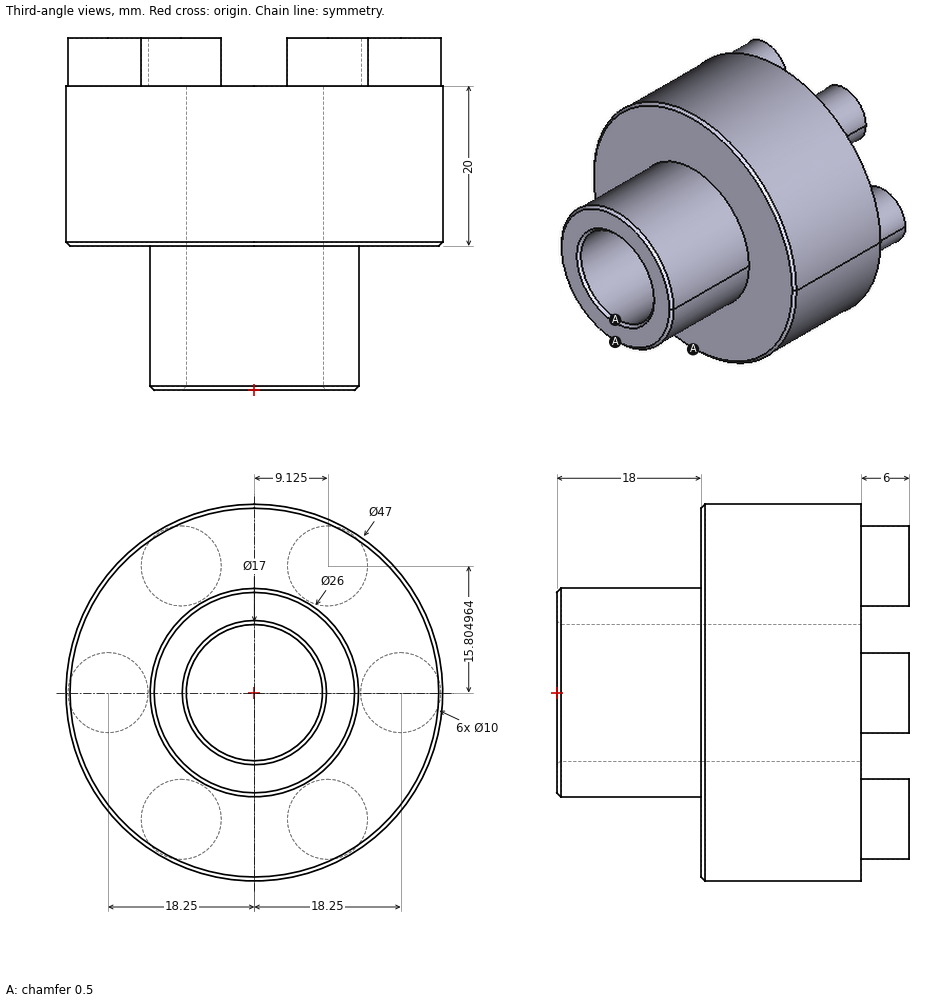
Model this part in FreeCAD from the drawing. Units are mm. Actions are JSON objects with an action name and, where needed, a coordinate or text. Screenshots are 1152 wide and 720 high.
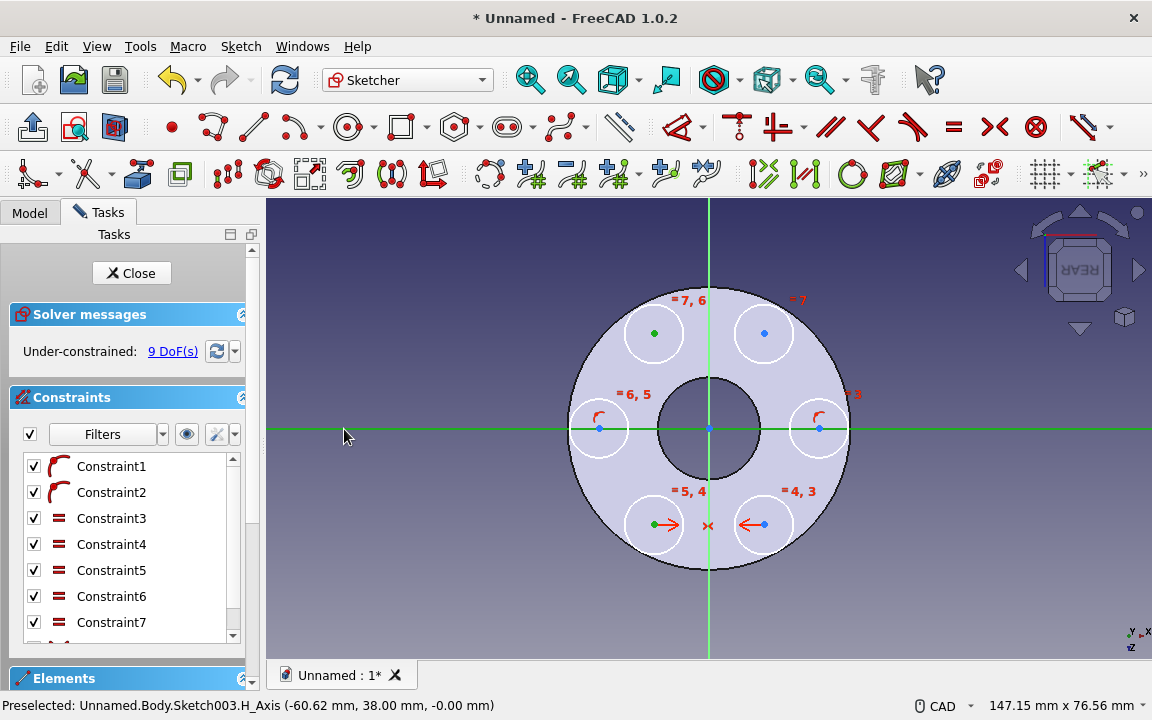
{"action": "left_click", "coordinate": [995, 128]}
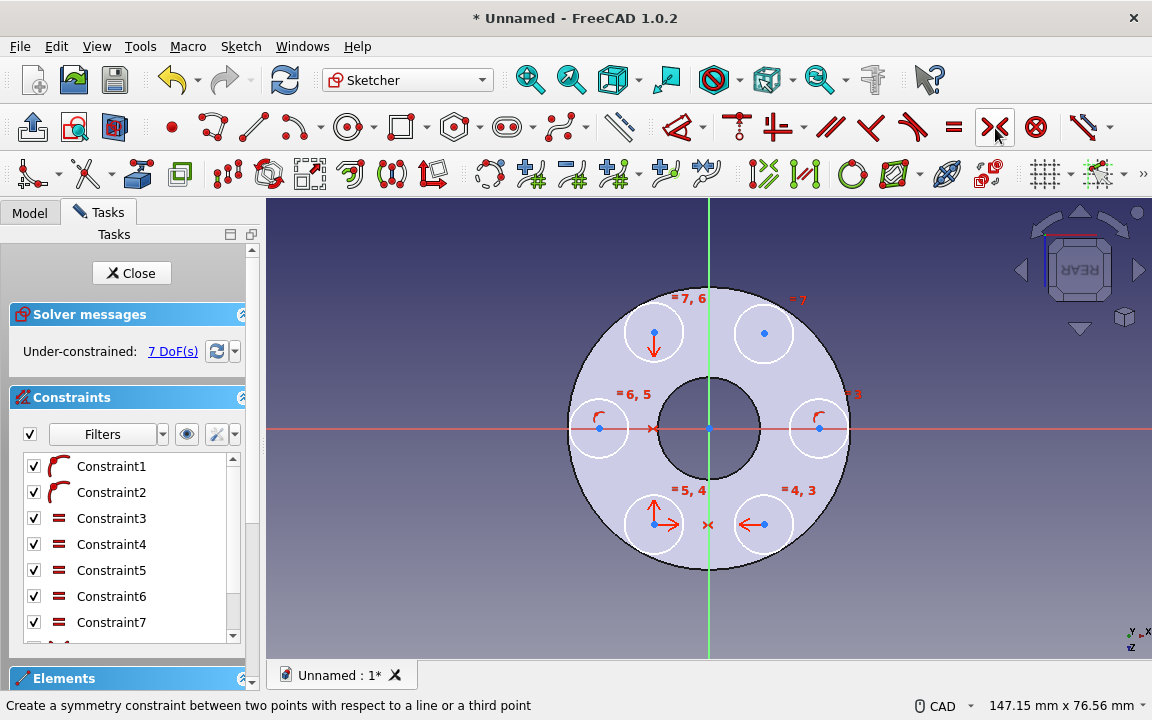
{"action": "left_click", "coordinate": [764, 525]}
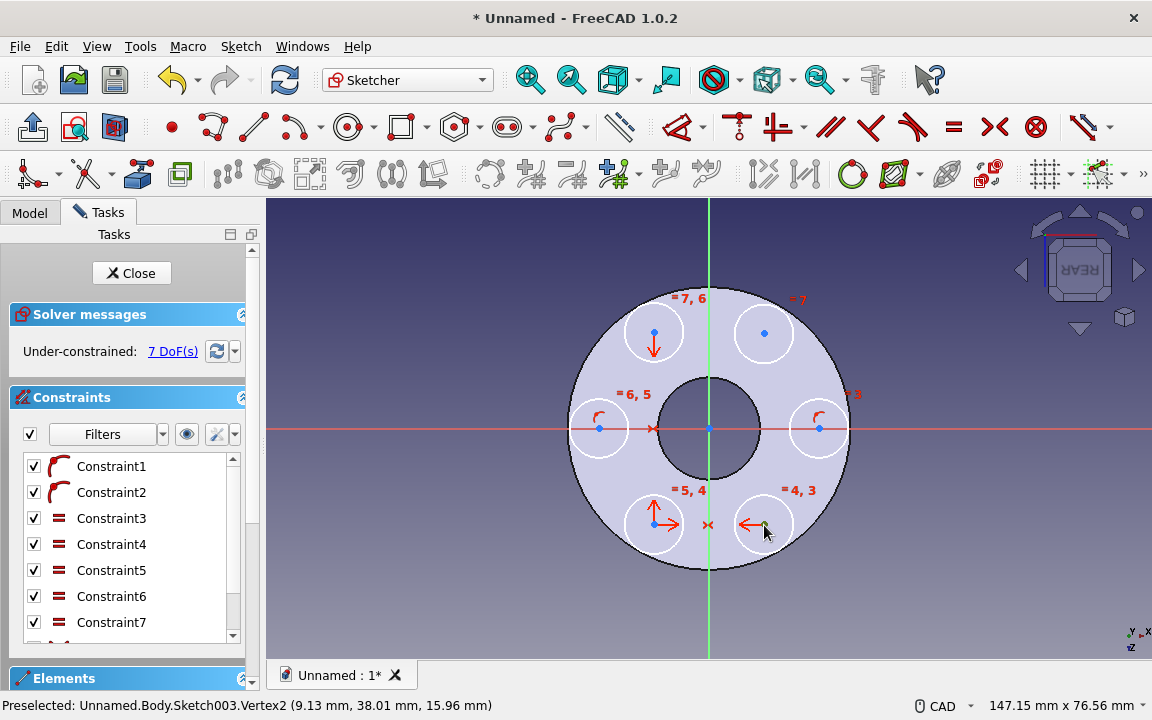
{"action": "left_click", "coordinate": [764, 334]}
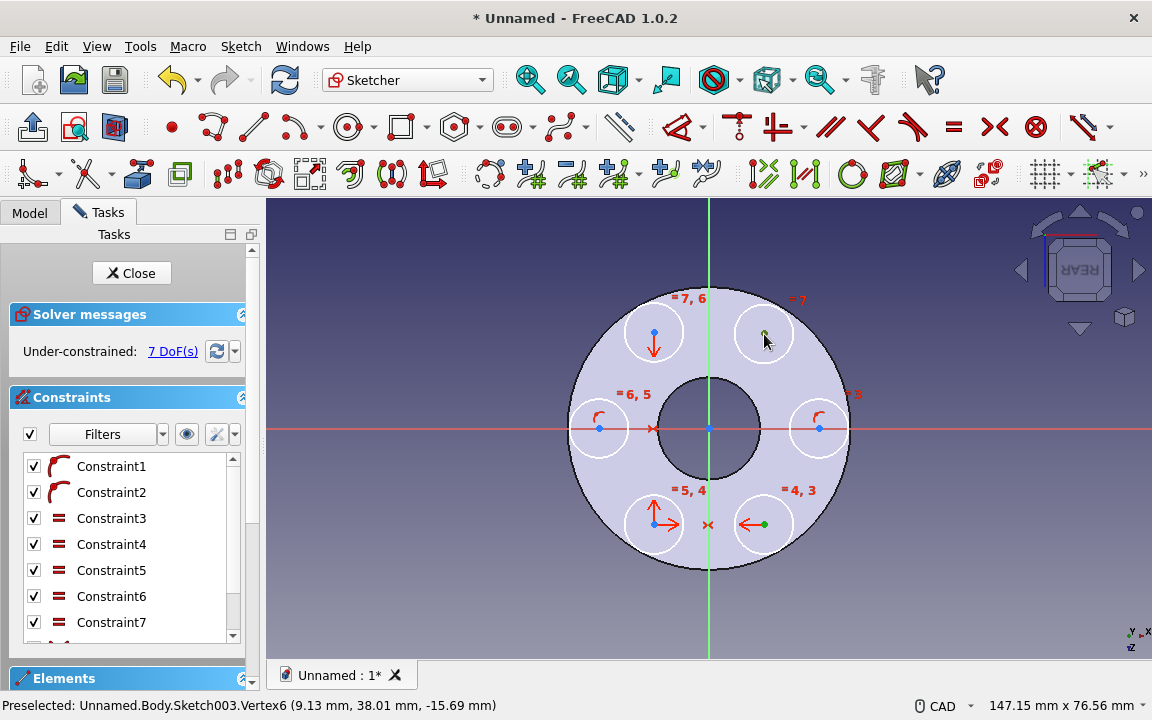
{"action": "left_click", "coordinate": [344, 429]}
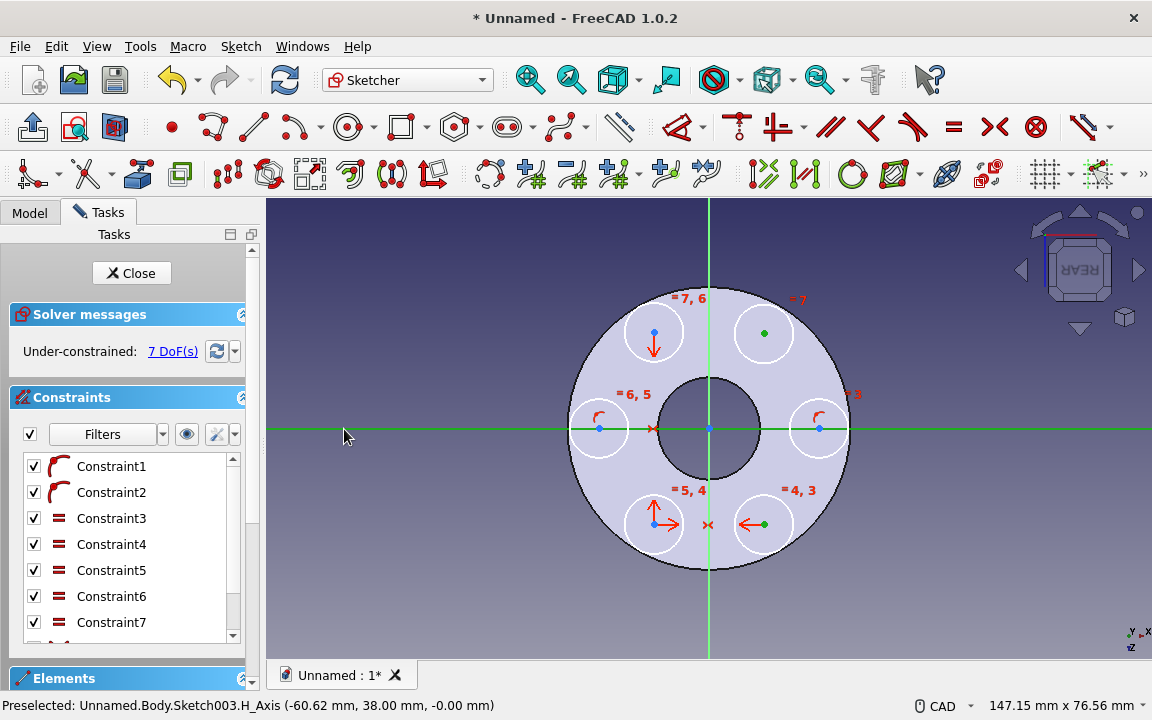
{"action": "left_click", "coordinate": [995, 128]}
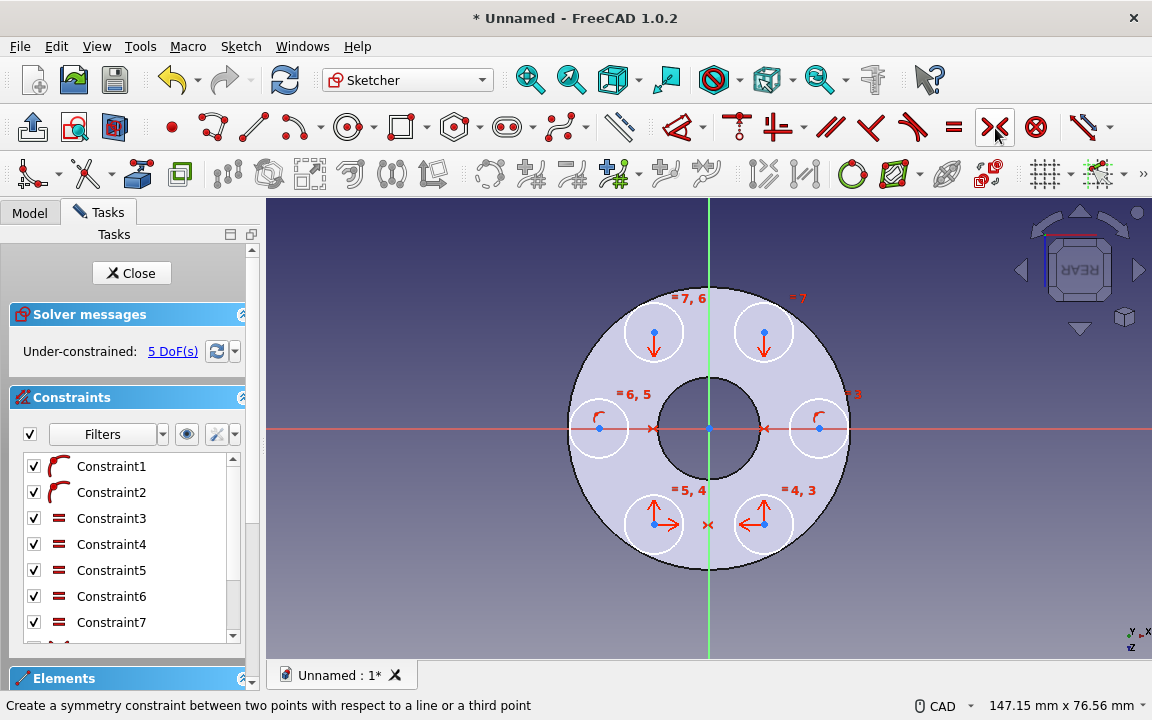
{"action": "left_click", "coordinate": [676, 128]}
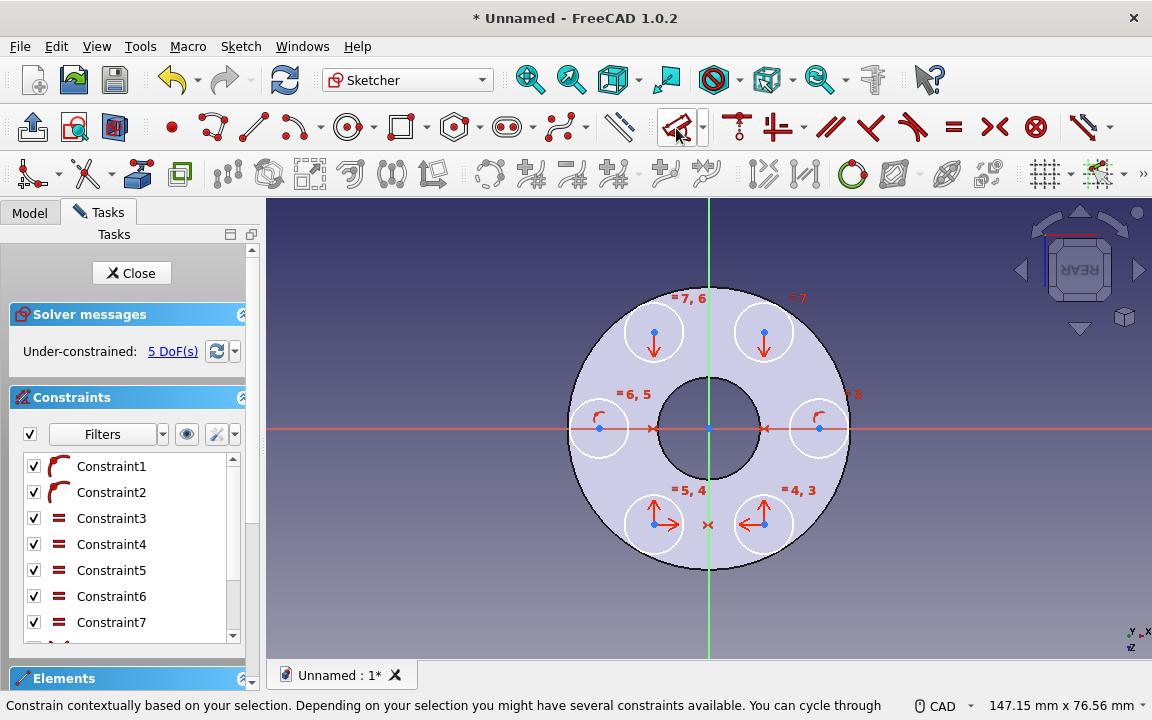
{"action": "left_click", "coordinate": [840, 408]}
{"action": "left_click", "coordinate": [863, 386]}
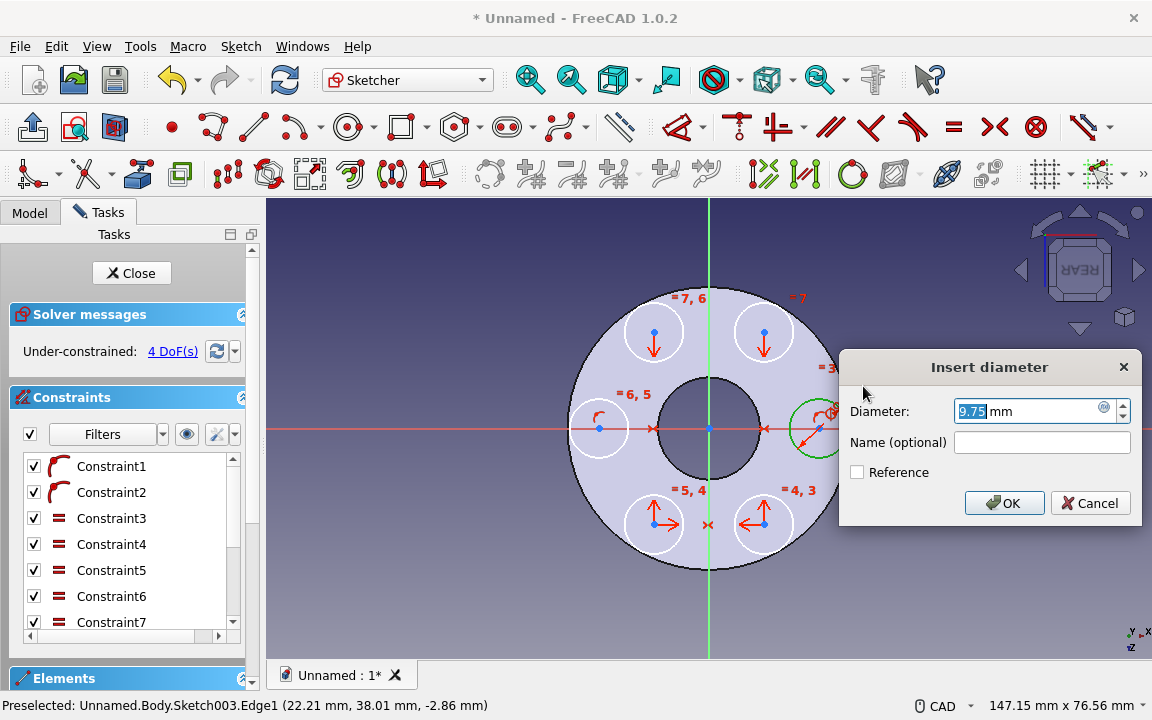
{"action": "type", "text": "10"}
{"action": "key", "text": "Return"}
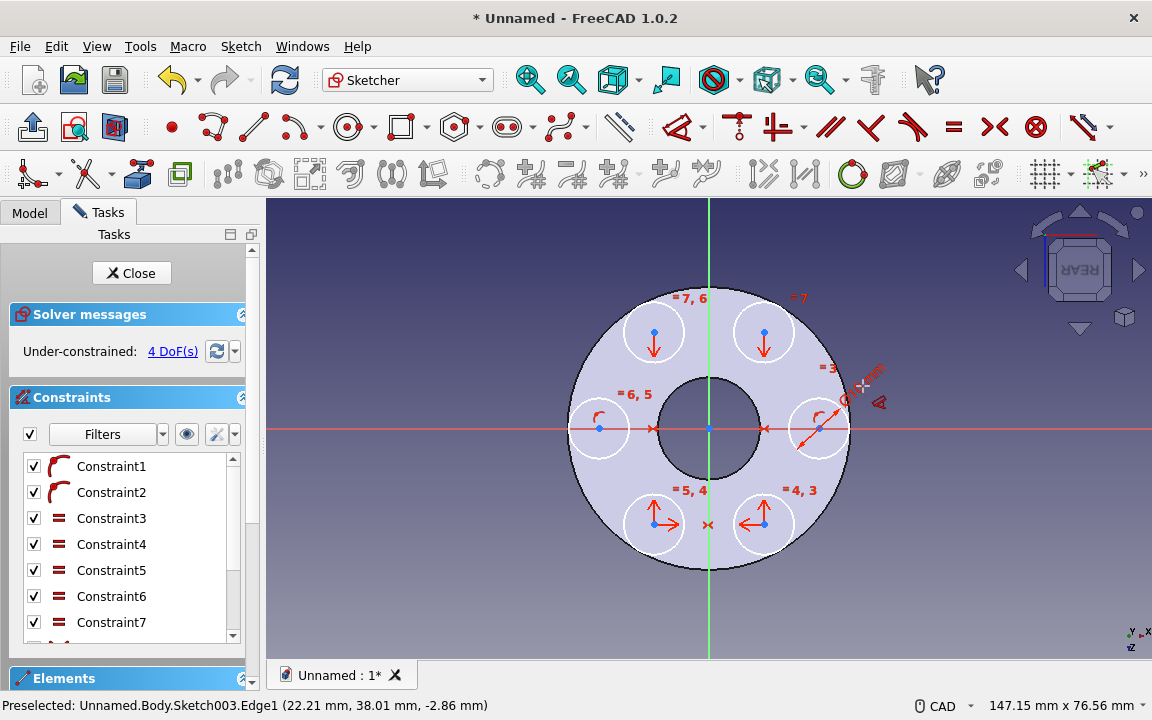
{"action": "left_click", "coordinate": [819, 429]}
{"action": "left_click", "coordinate": [764, 463]}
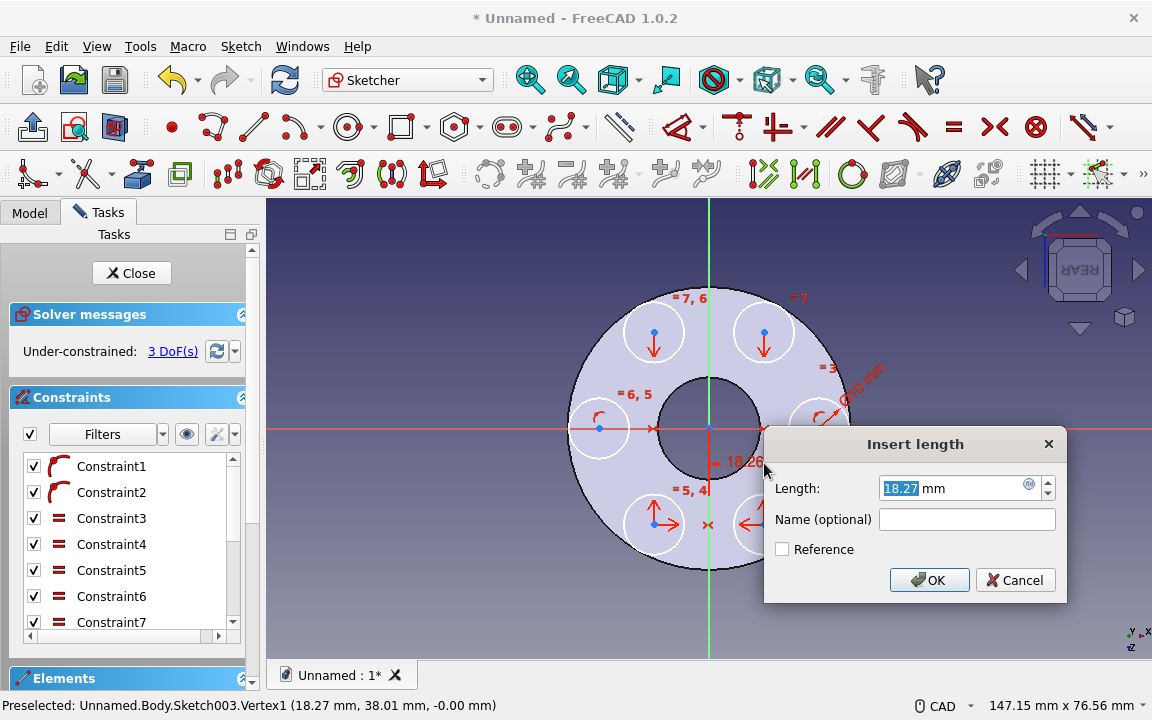
{"action": "type", "text": "18.25"}
{"action": "key", "text": "Return"}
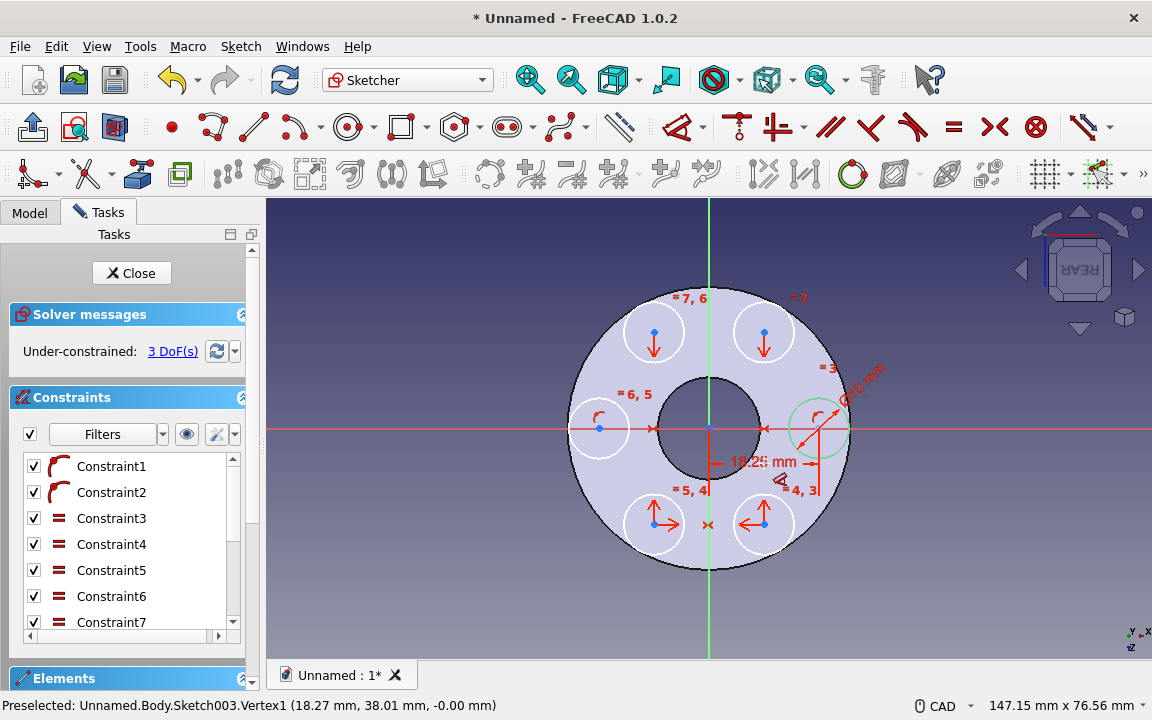
{"action": "left_click", "coordinate": [764, 525]}
{"action": "left_click", "coordinate": [736, 559]}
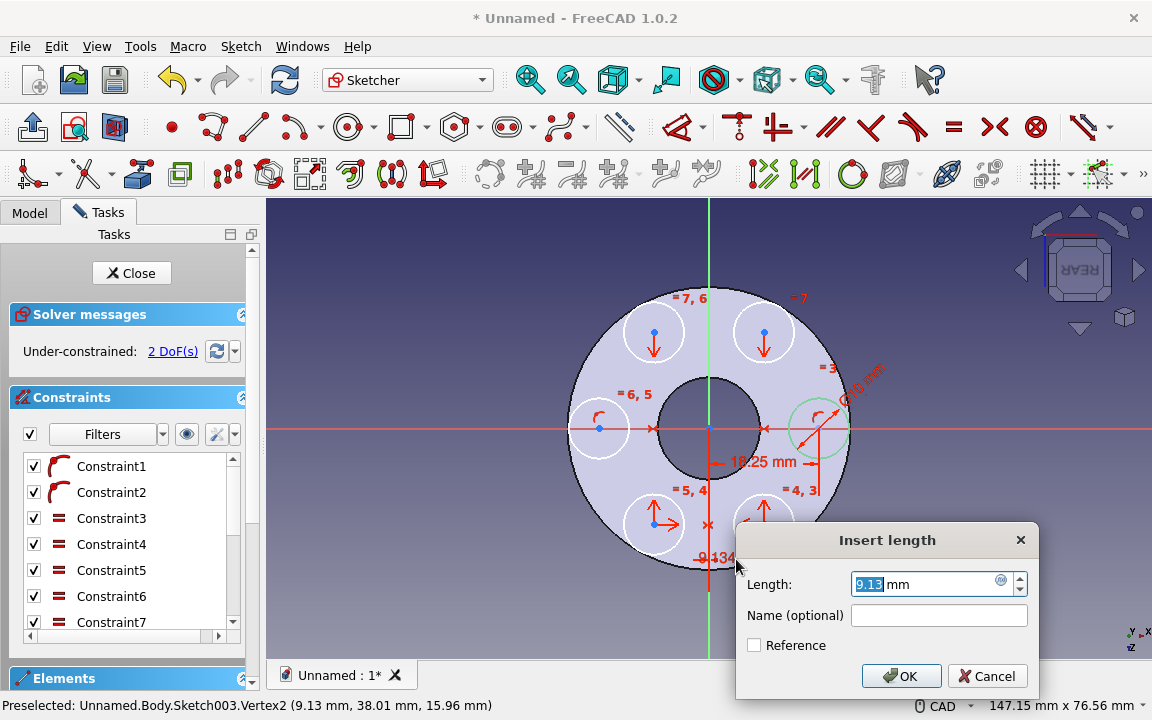
{"action": "type", "text": "9.125"}
{"action": "key", "text": "Return"}